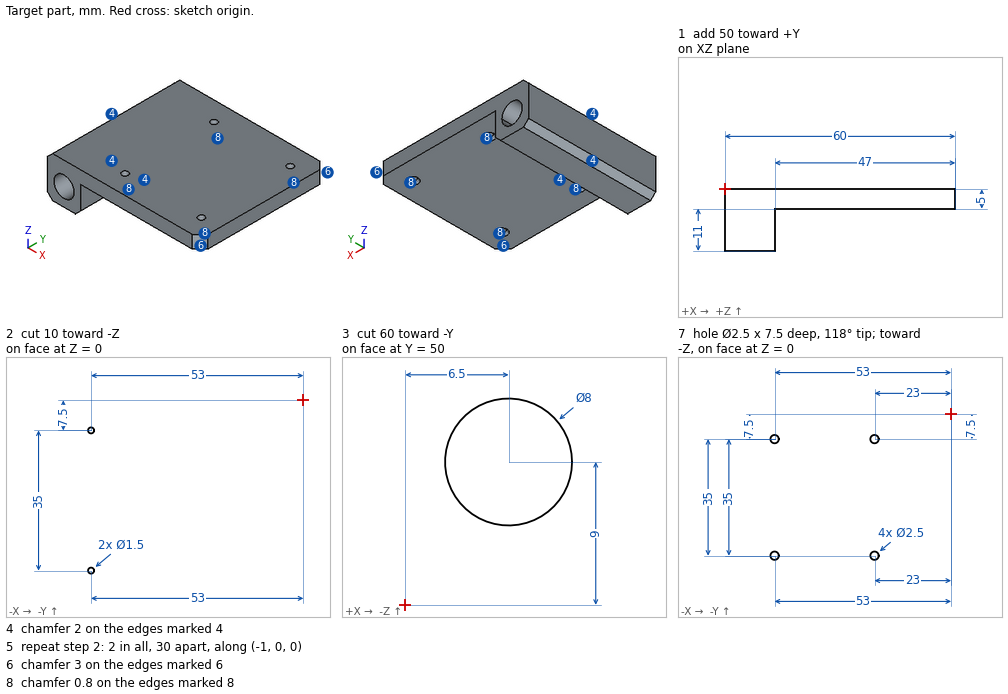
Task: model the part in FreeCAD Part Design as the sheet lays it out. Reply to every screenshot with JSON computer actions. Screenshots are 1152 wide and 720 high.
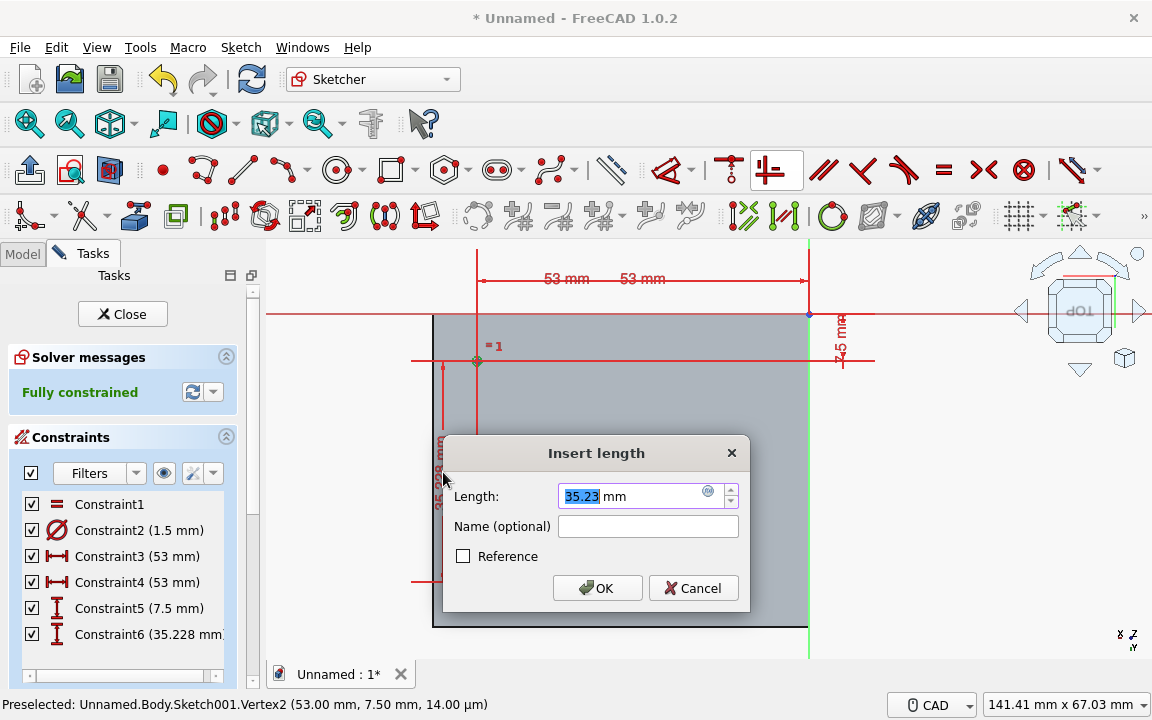
{"action": "type", "text": "35"}
{"action": "key", "text": "Return"}
{"action": "key", "text": "Escape"}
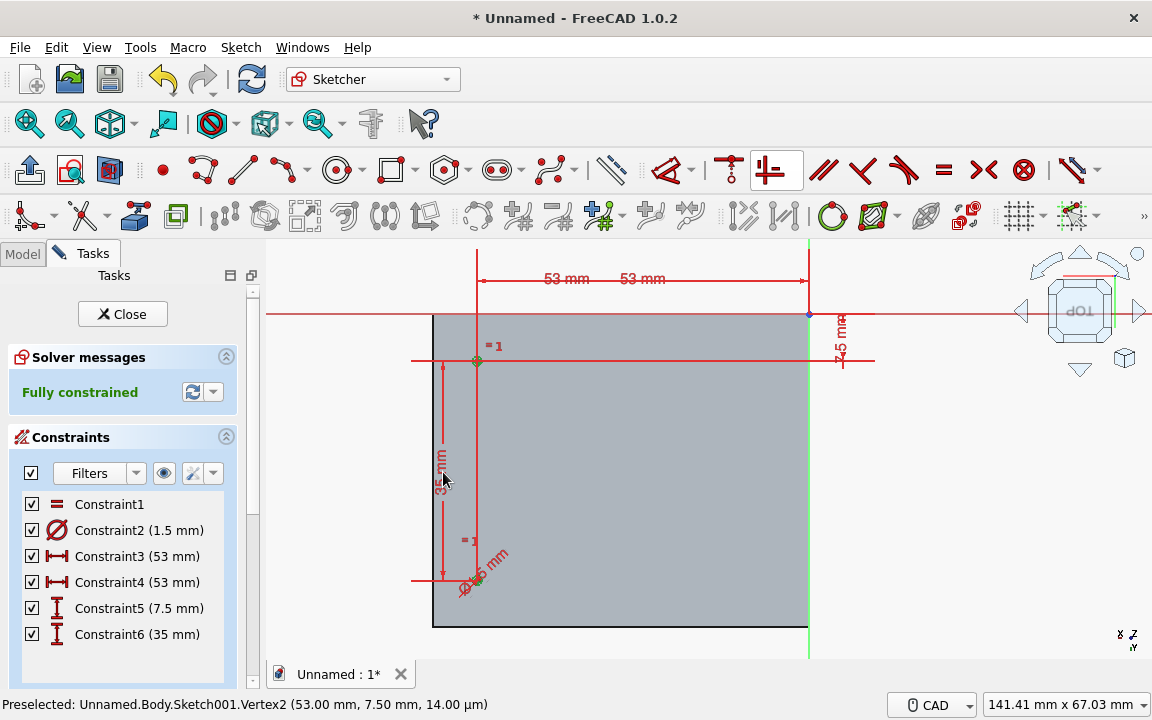
{"action": "left_click", "coordinate": [123, 314]}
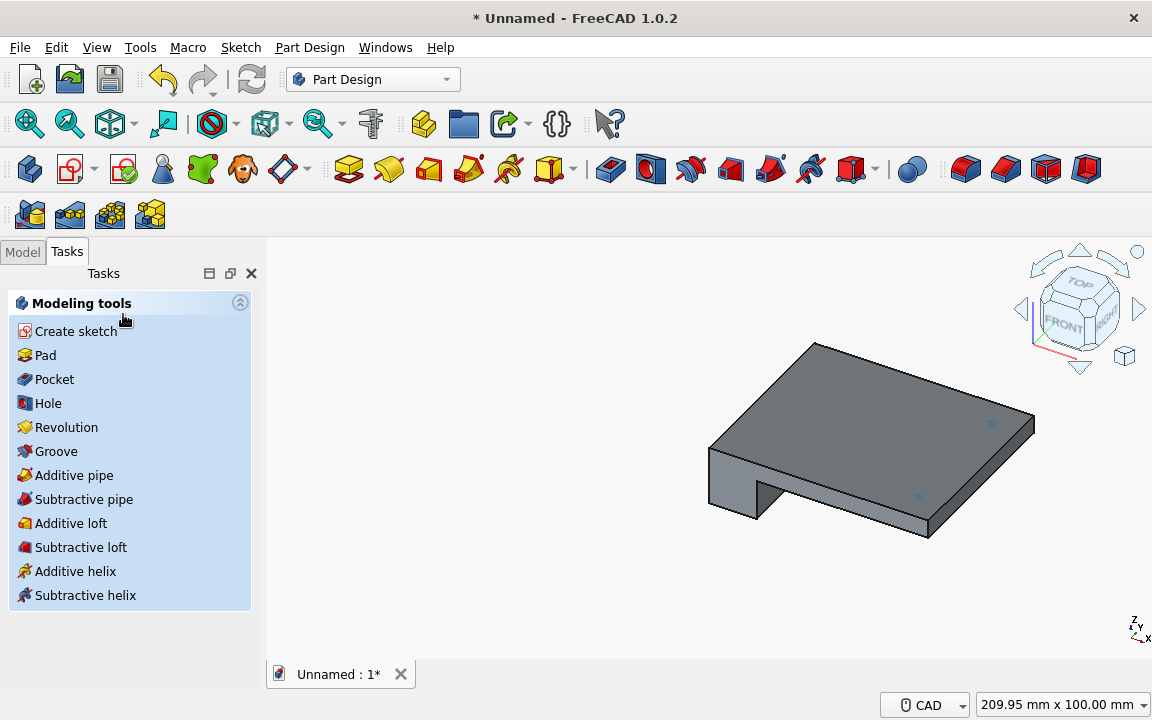
{"action": "left_click", "coordinate": [612, 170]}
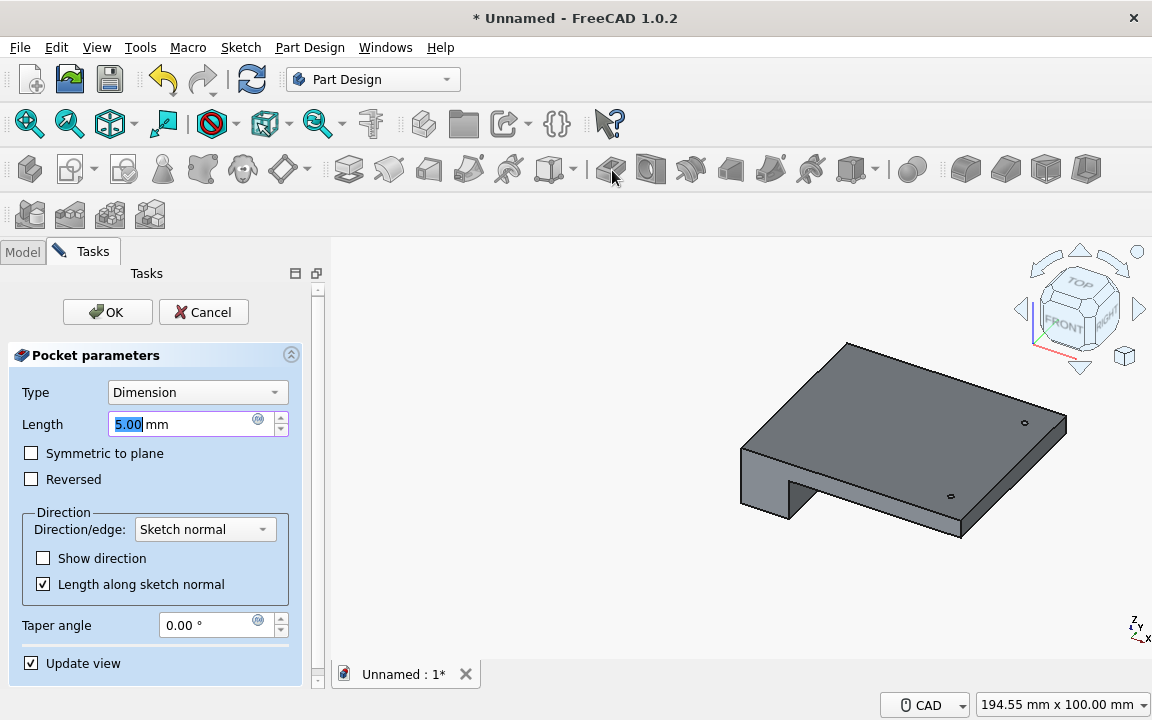
{"action": "type", "text": "10"}
{"action": "key", "text": "Tab"}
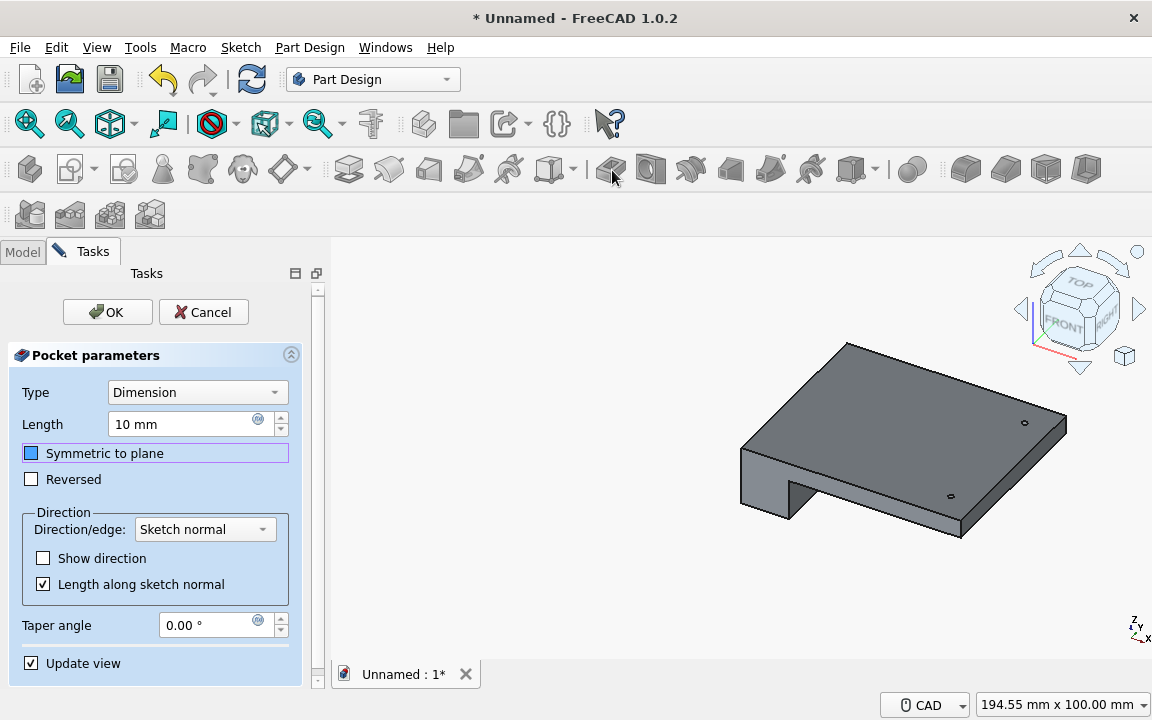
{"action": "left_click", "coordinate": [108, 312]}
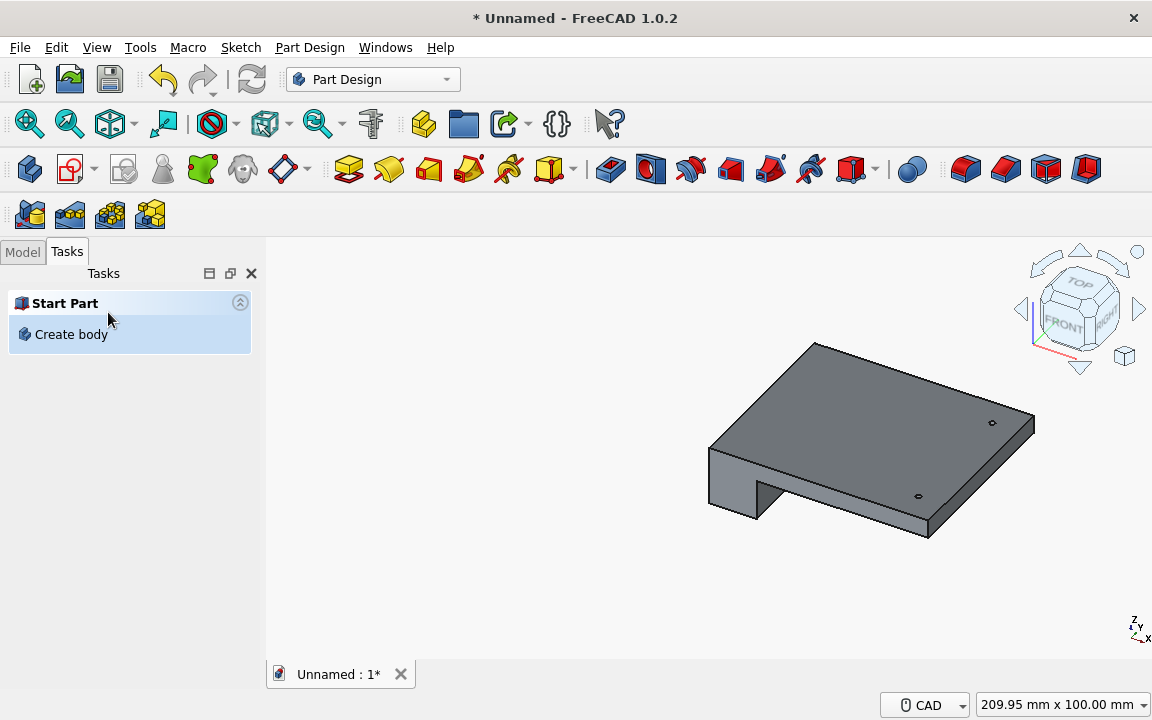
{"action": "key", "text": "4"}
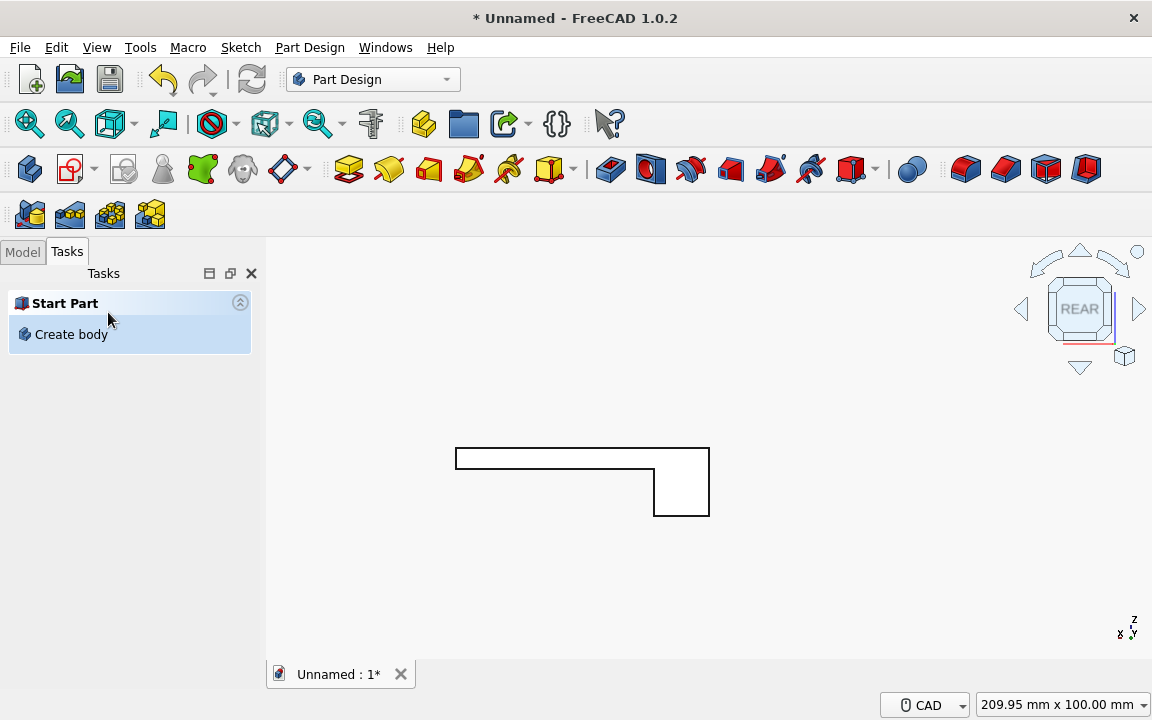
{"action": "key", "text": "v f"}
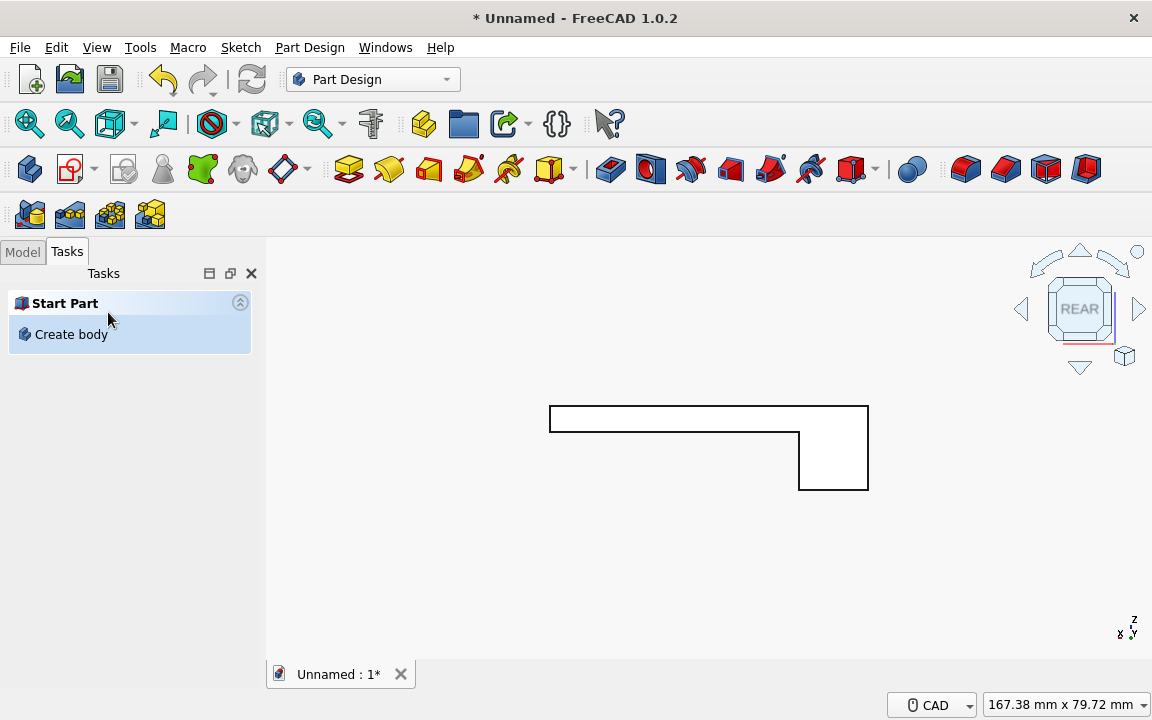
{"action": "left_click", "coordinate": [845, 435]}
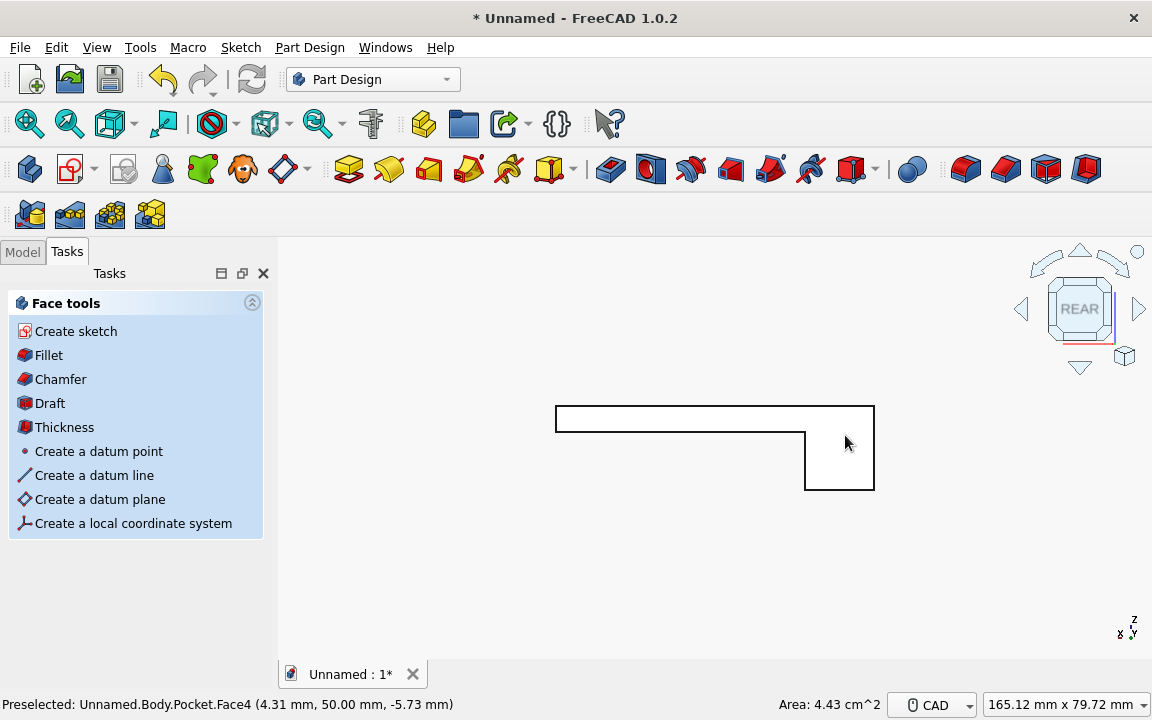
{"action": "left_click", "coordinate": [70, 170]}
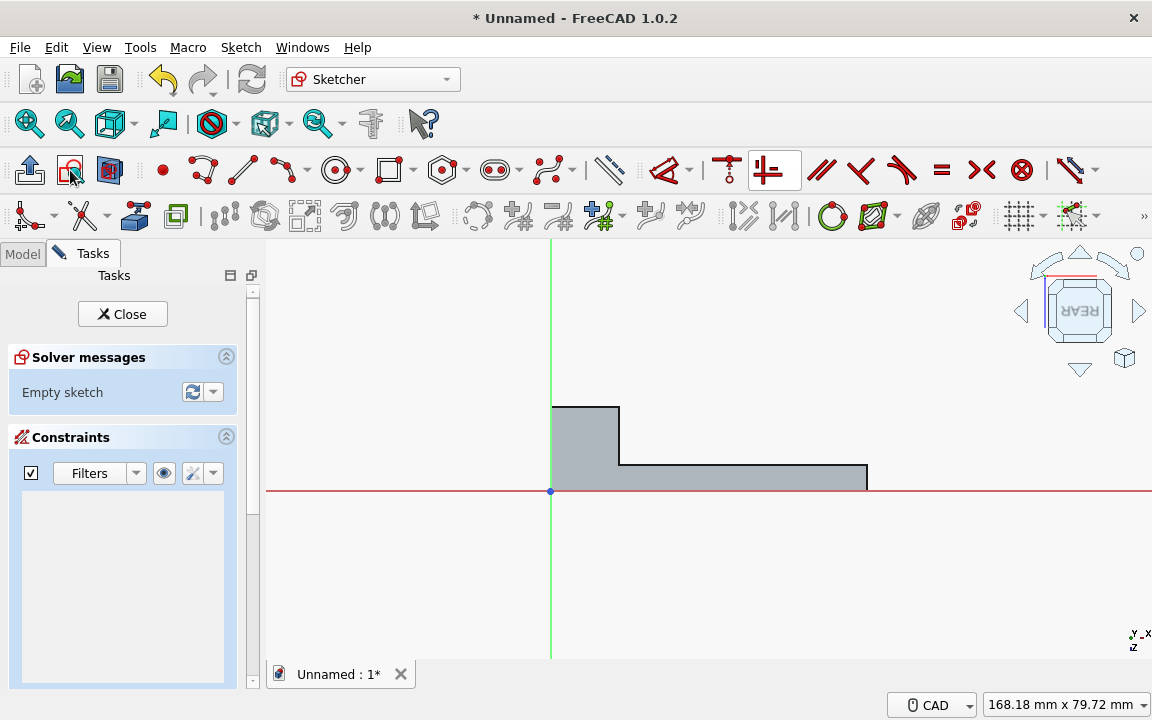
{"action": "scroll", "coordinate": [558, 459], "scroll_direction": "up", "scroll_amount": 7}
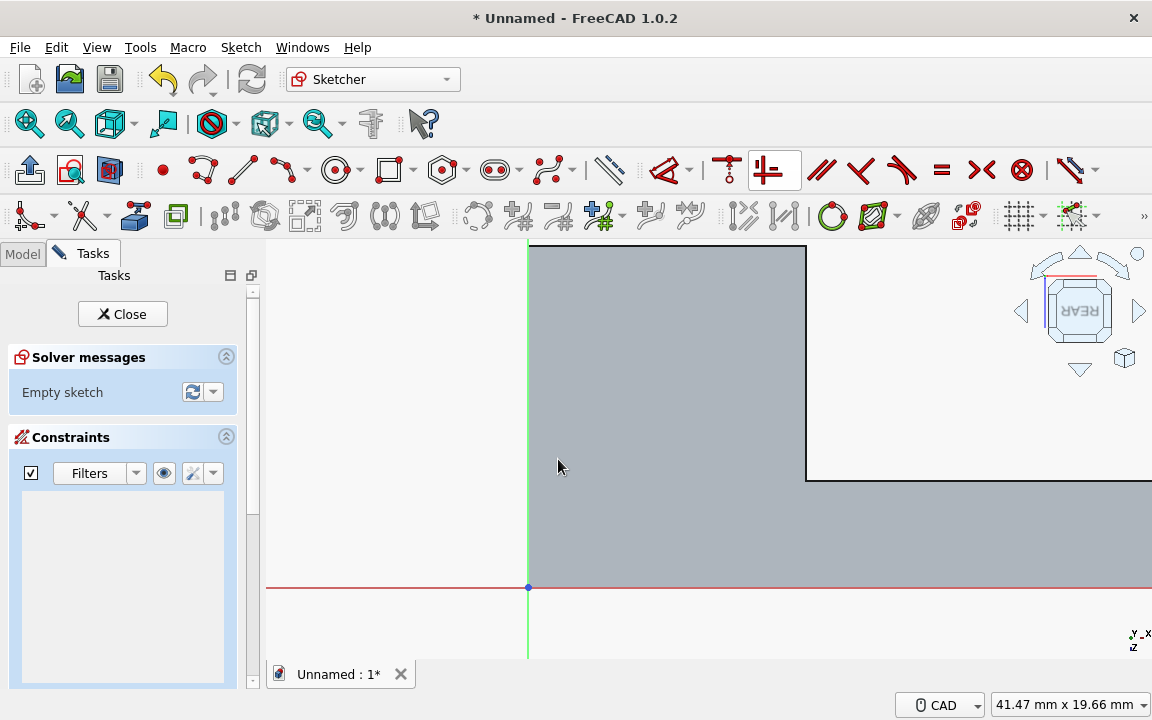
{"action": "left_click", "coordinate": [336, 170]}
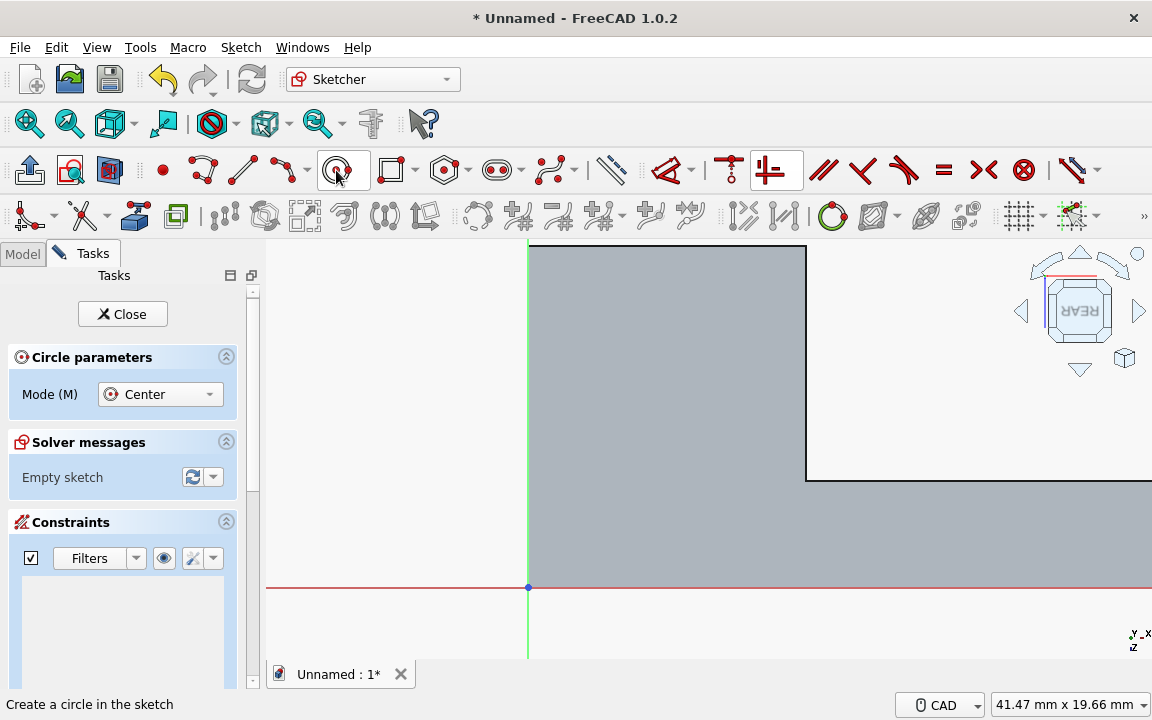
{"action": "left_click", "coordinate": [667, 395]}
{"action": "left_click", "coordinate": [728, 335]}
{"action": "key", "text": "Escape"}